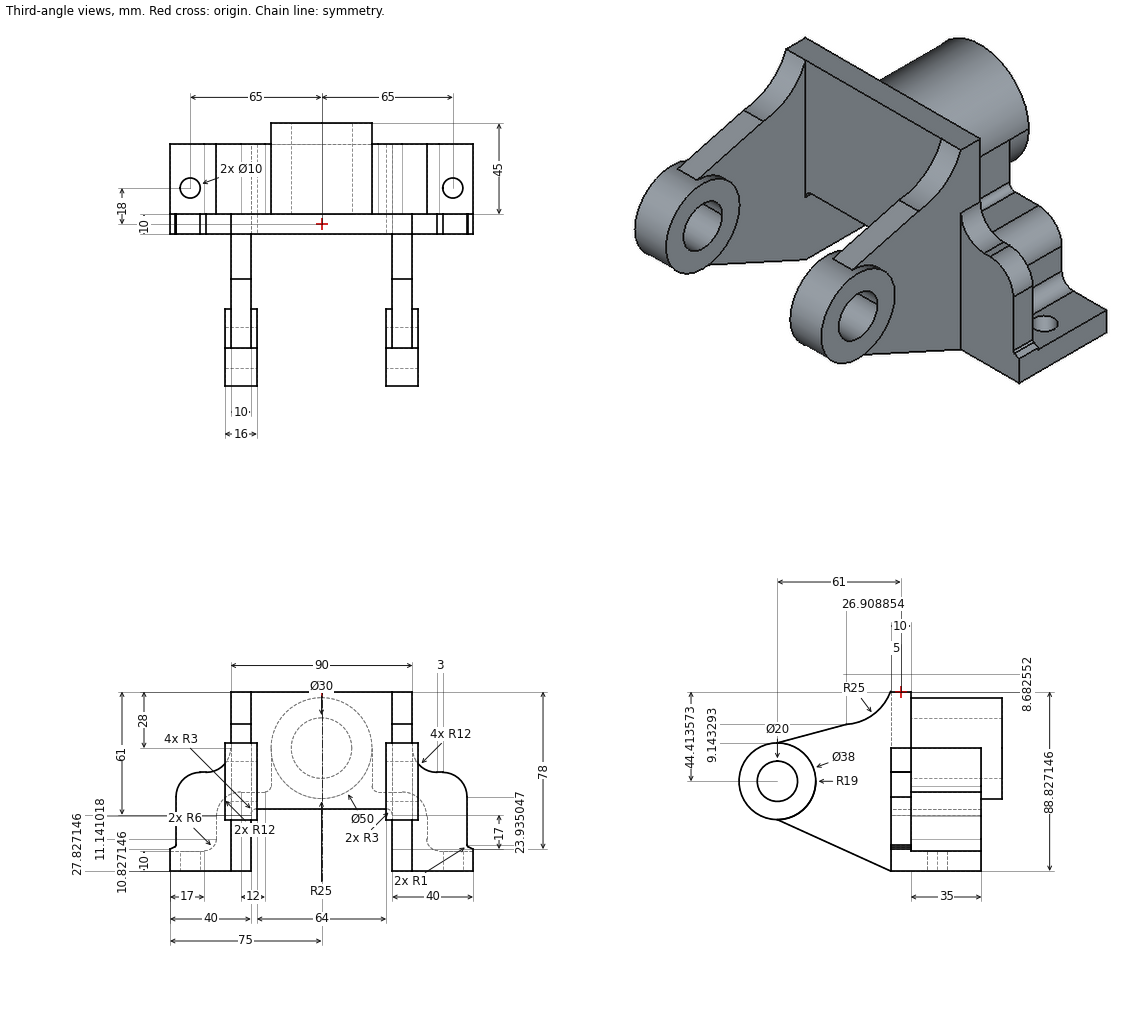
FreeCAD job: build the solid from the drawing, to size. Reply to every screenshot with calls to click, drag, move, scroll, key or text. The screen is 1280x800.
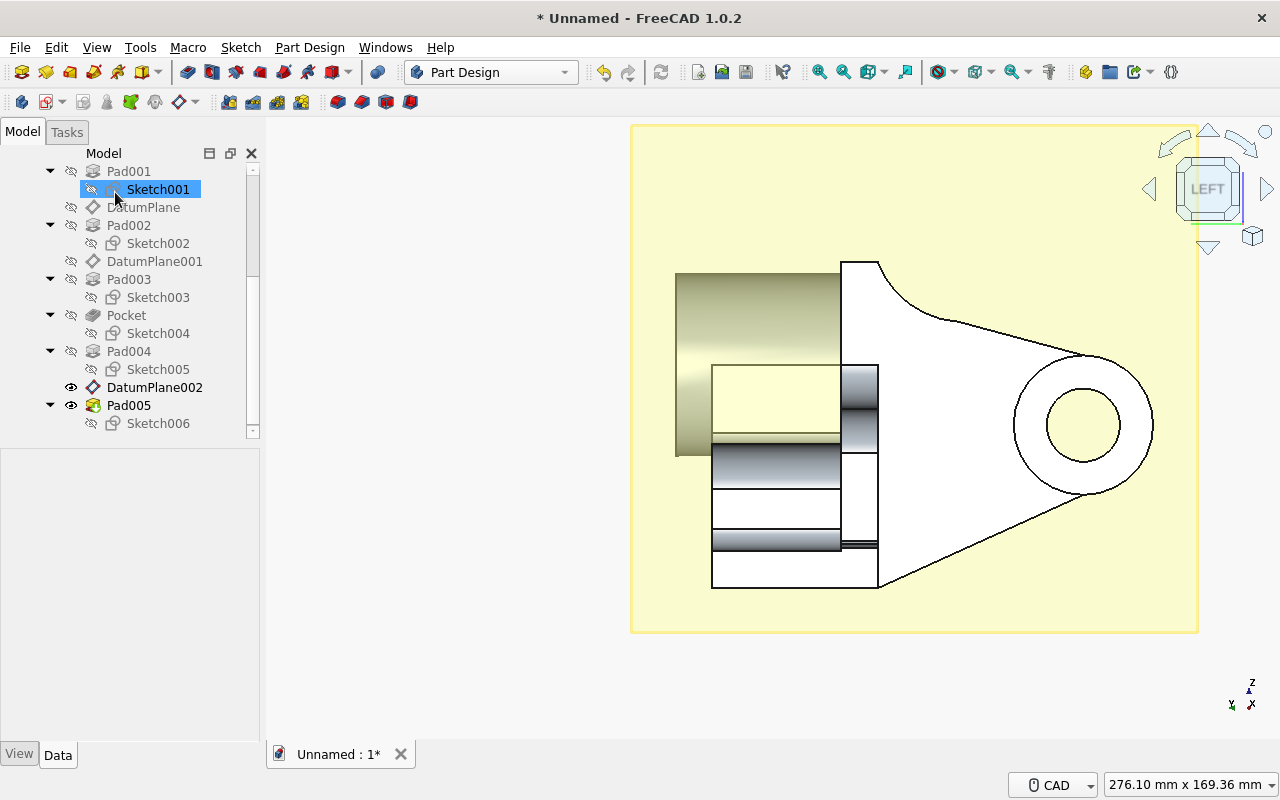
click(116, 387)
key(space)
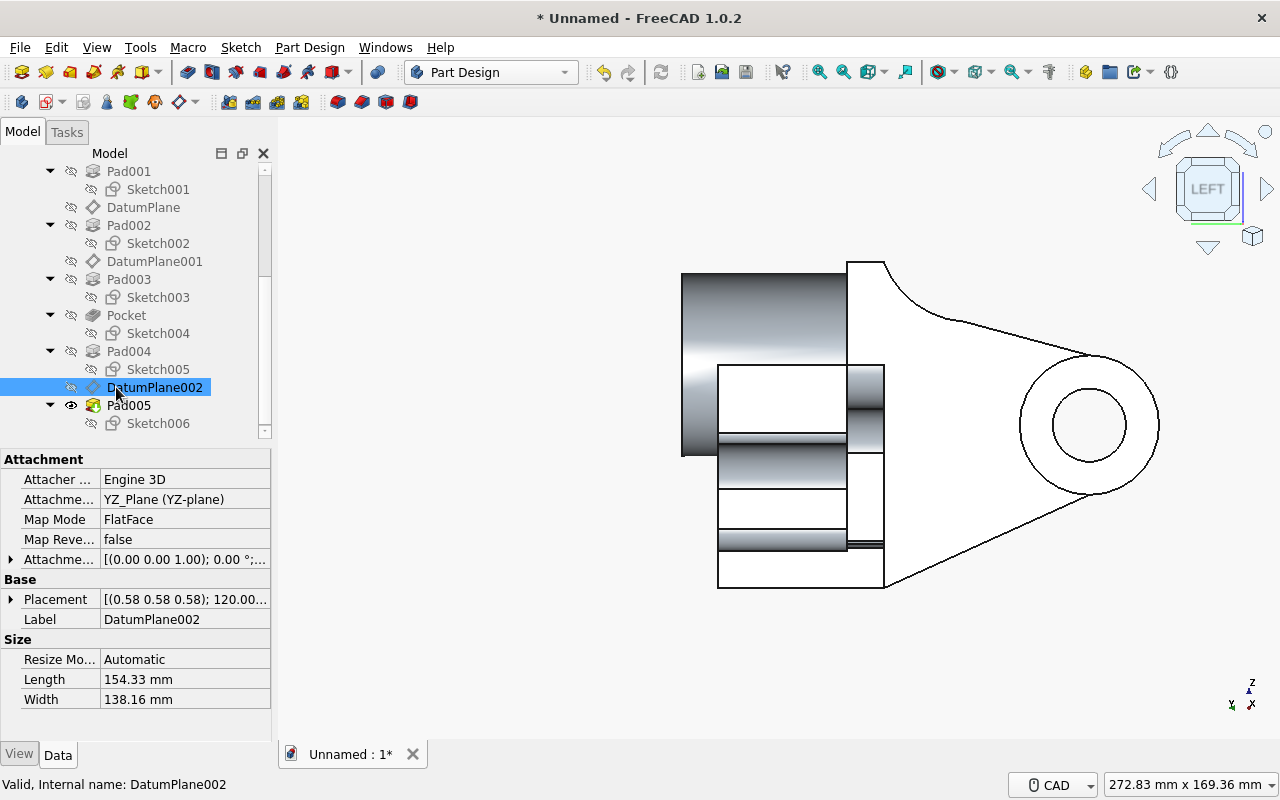
click(116, 351)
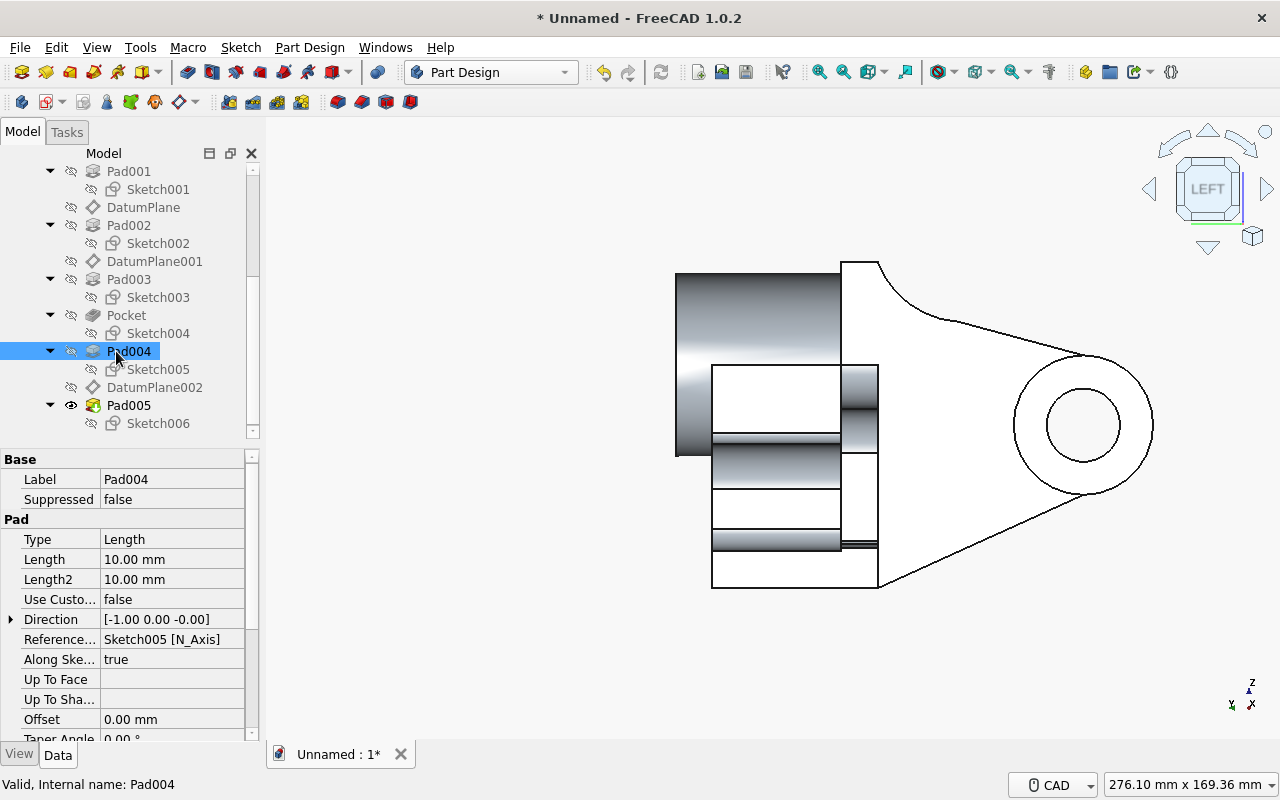
click(116, 405, ctrl)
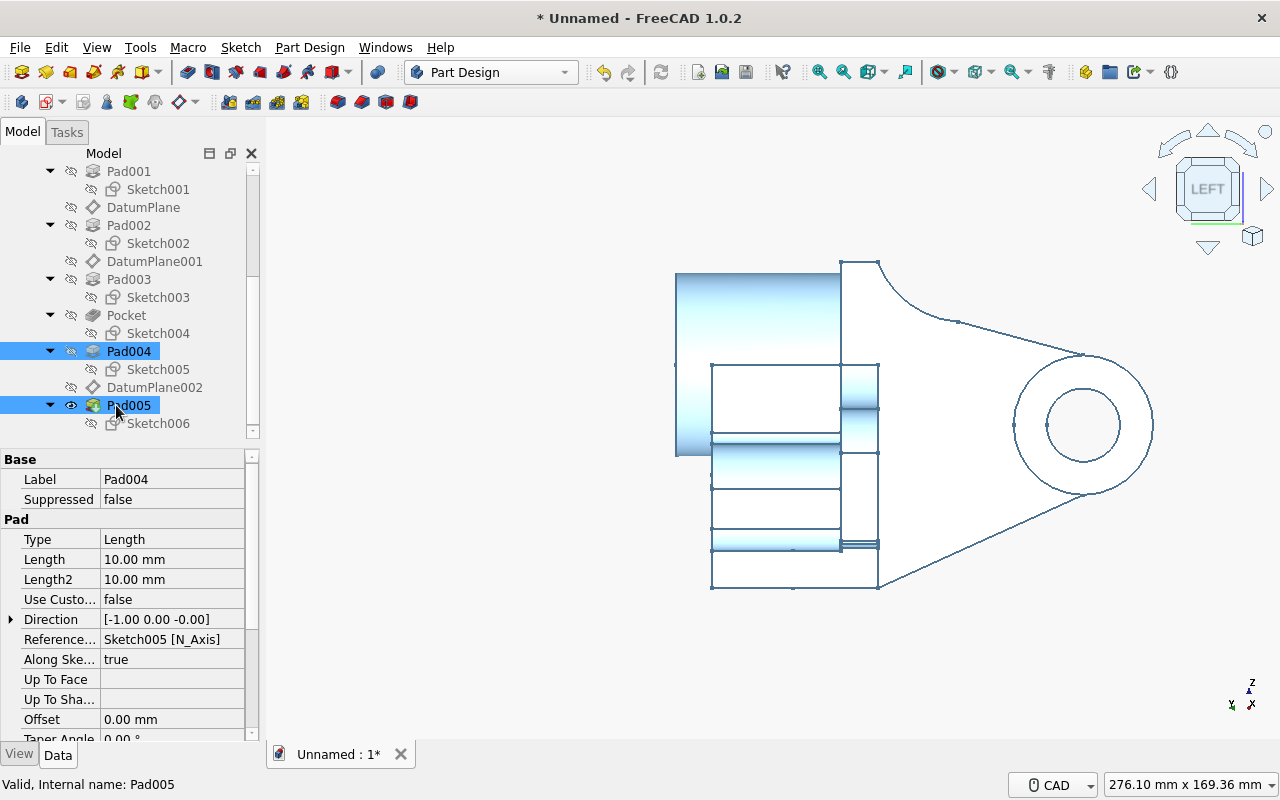
click(230, 102)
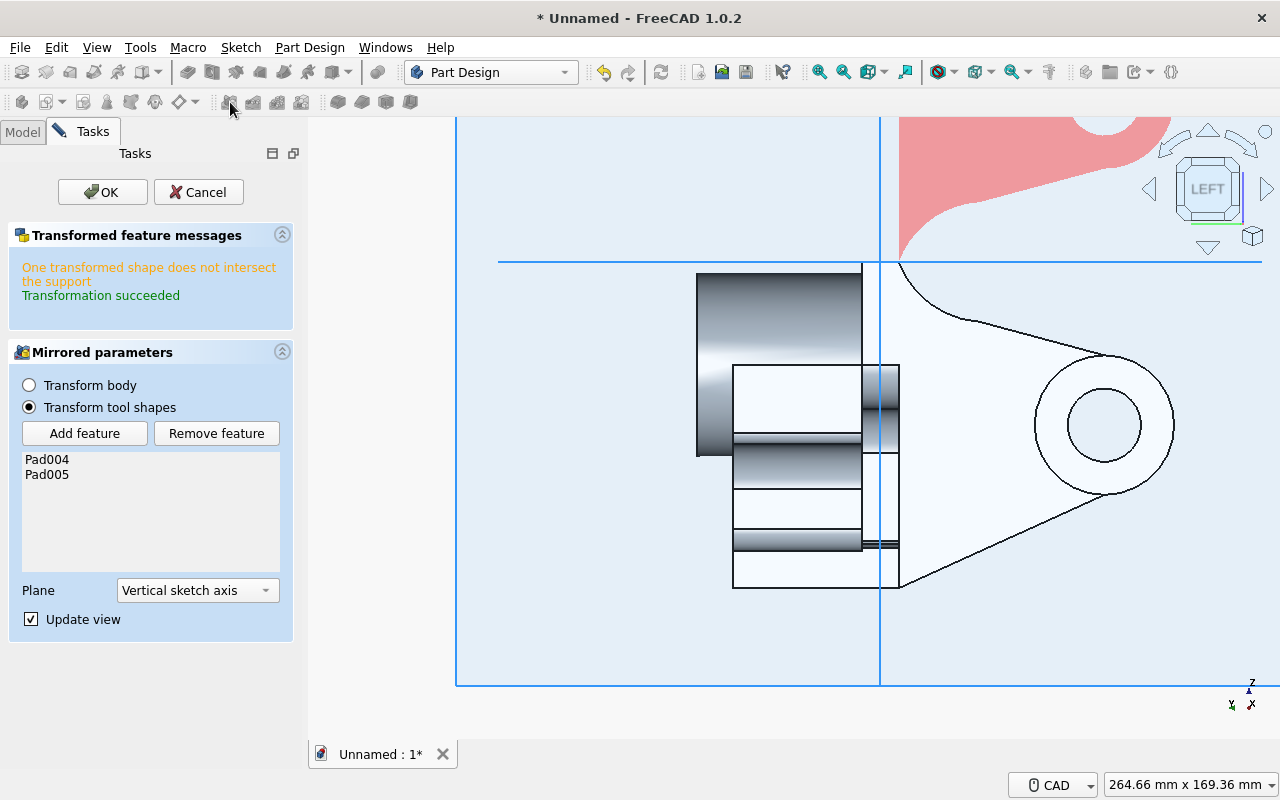
click(198, 590)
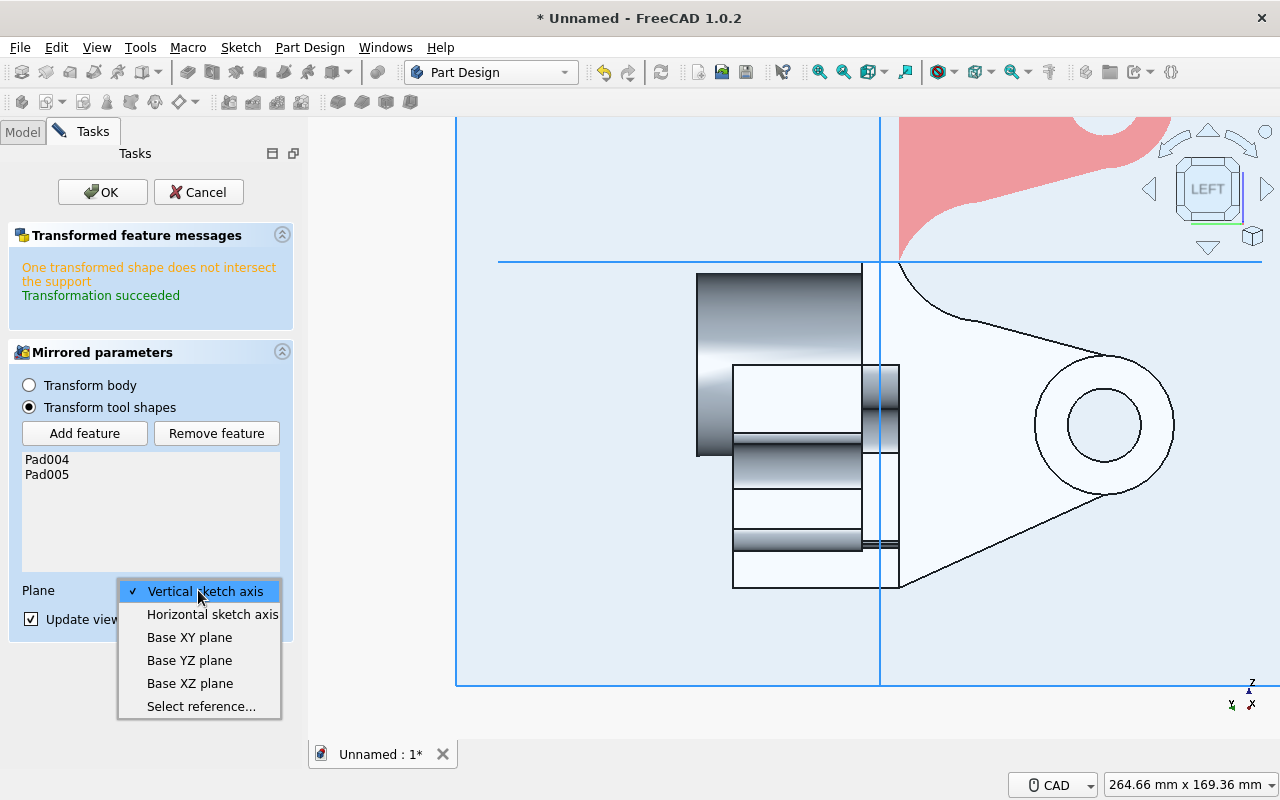
click(198, 660)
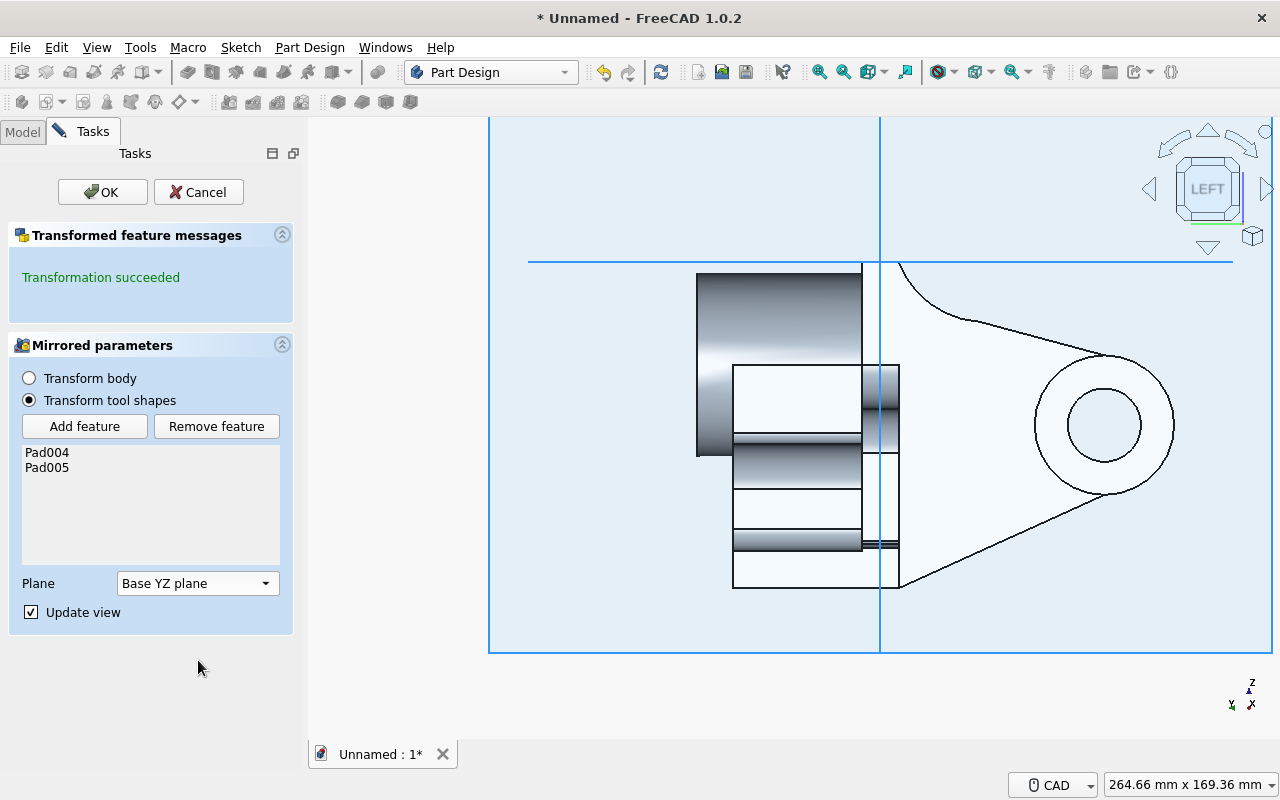
click(103, 192)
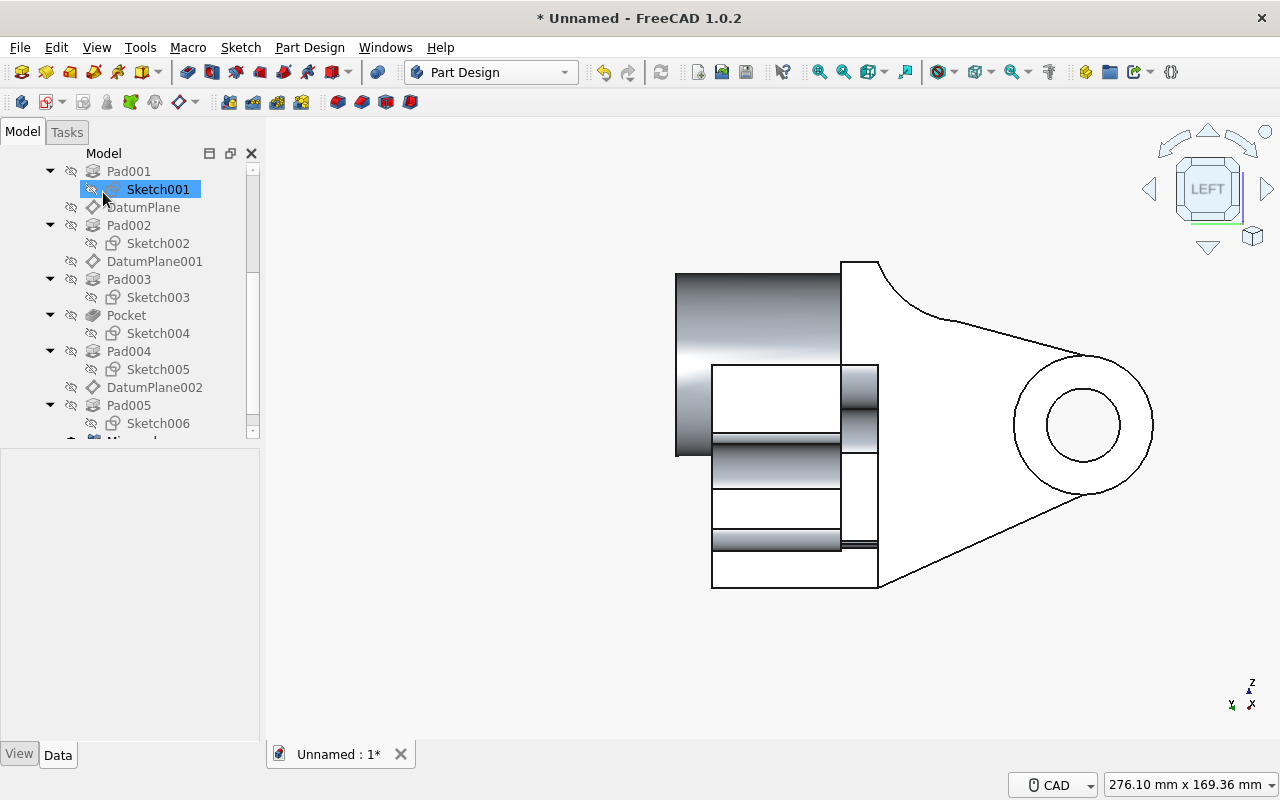
key(0)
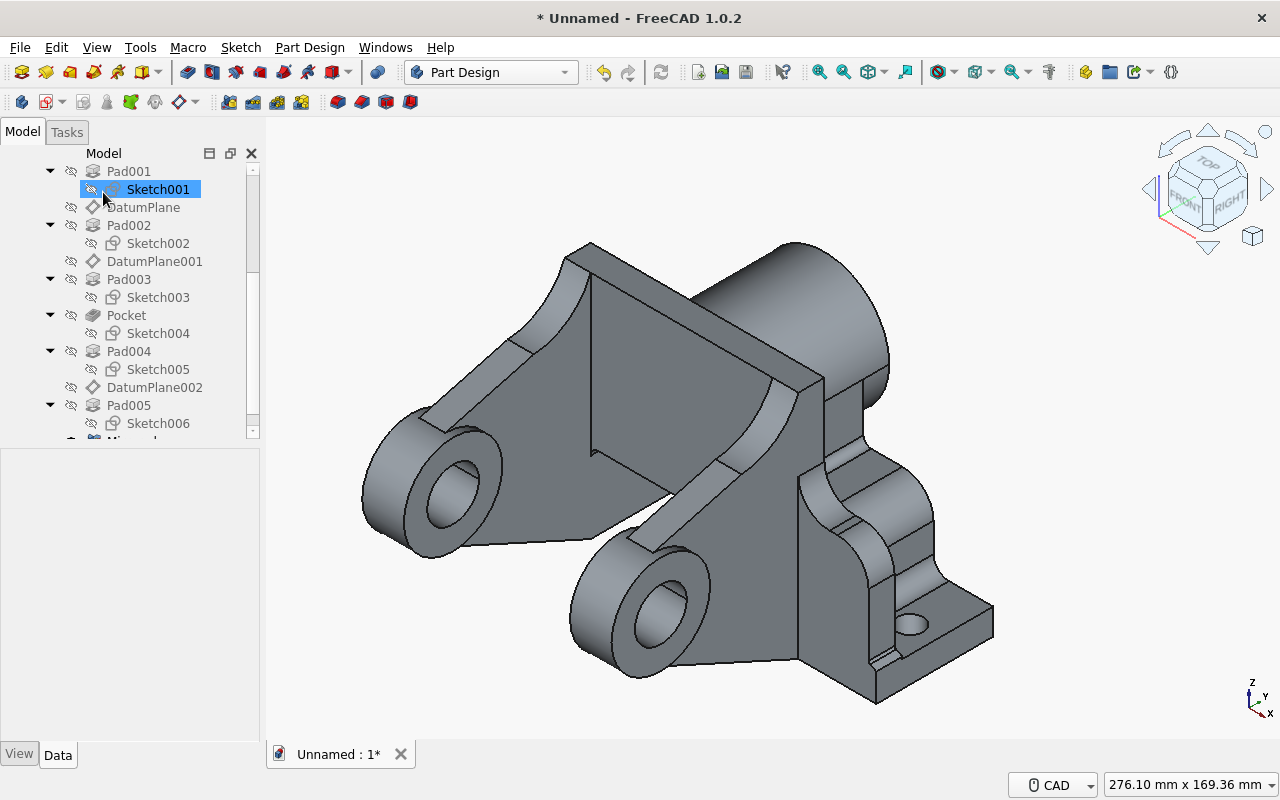
key(v)
key(f)